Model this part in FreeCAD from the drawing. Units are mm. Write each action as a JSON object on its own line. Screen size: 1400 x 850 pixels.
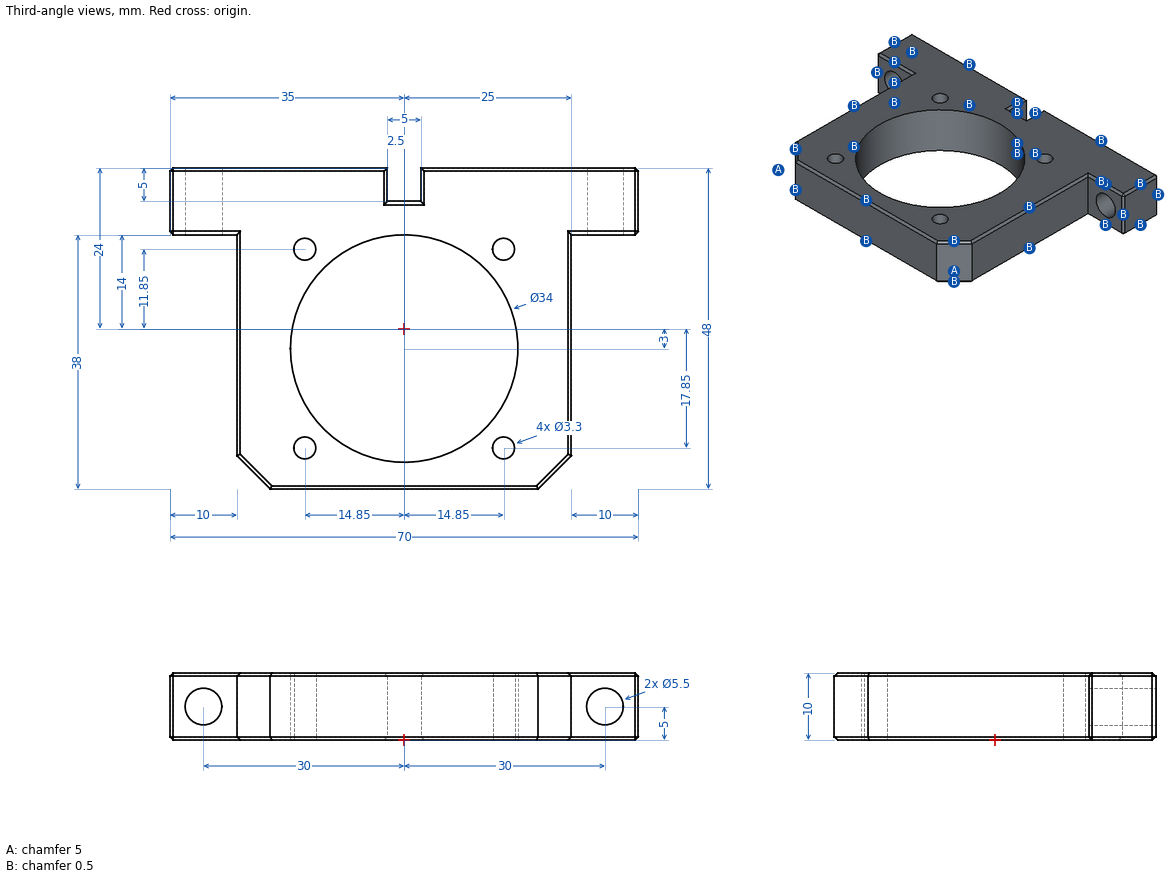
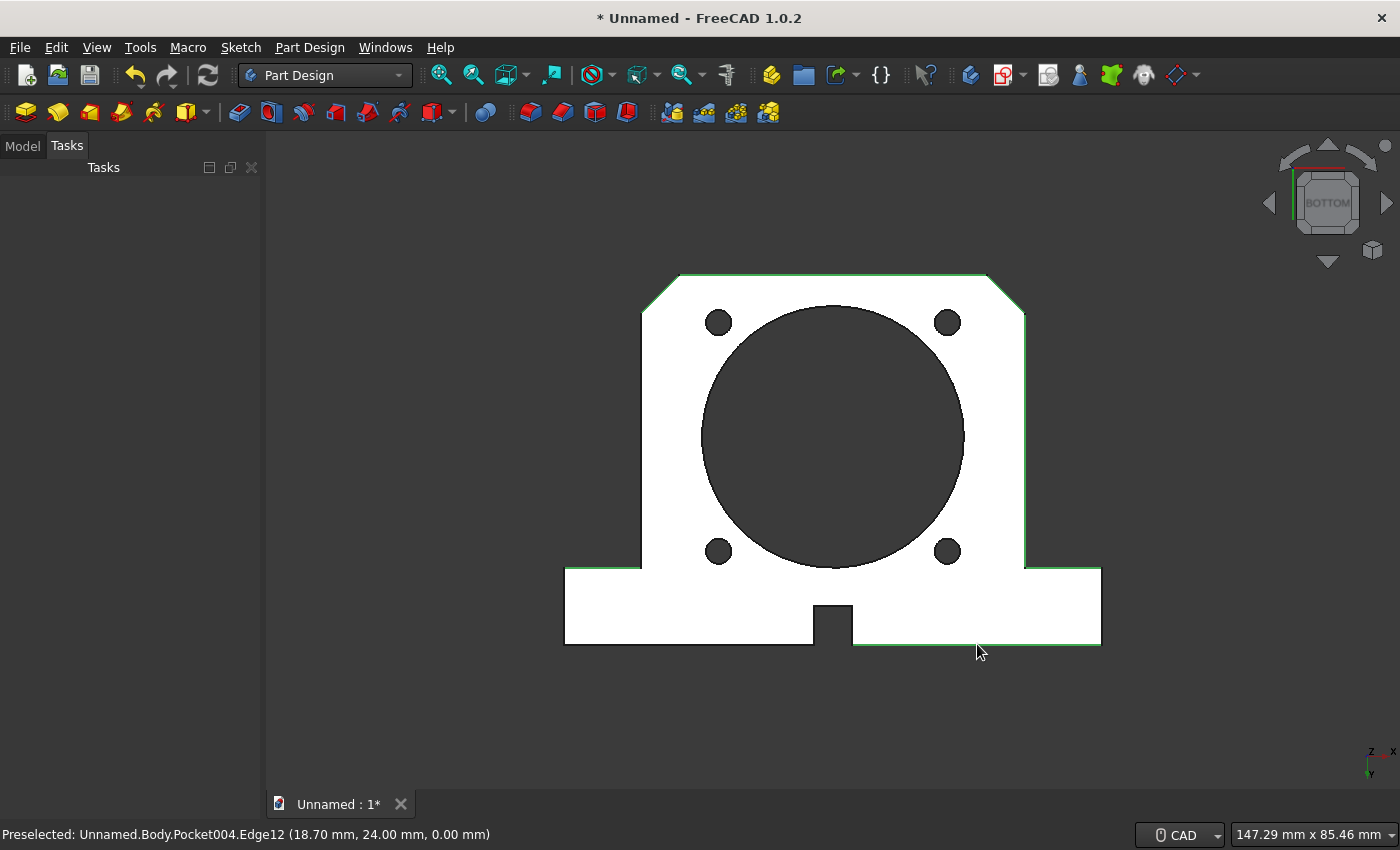
{"action": "left_click", "coordinate": [641, 440], "text": "ctrl"}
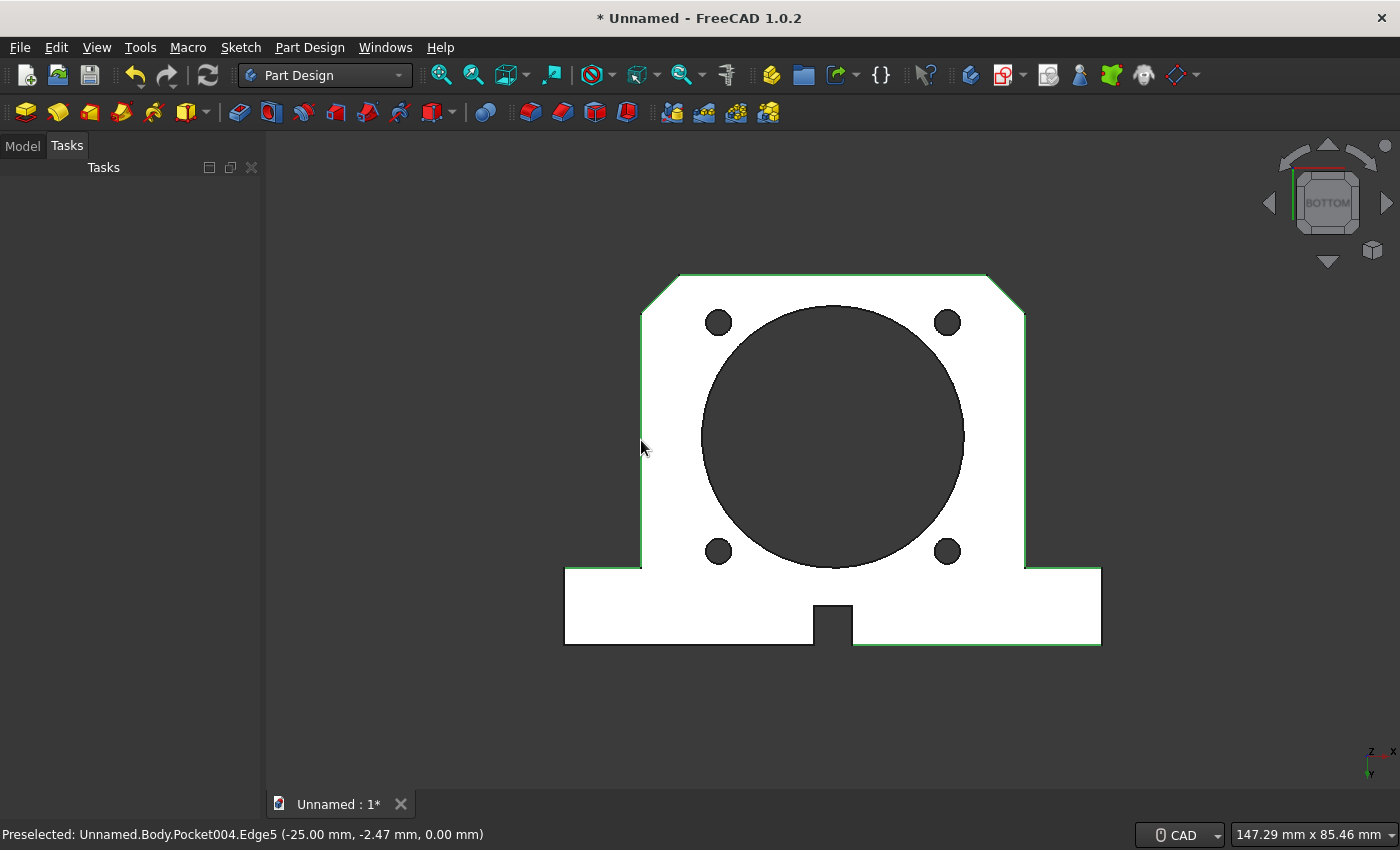
{"action": "left_click", "coordinate": [689, 644], "text": "ctrl"}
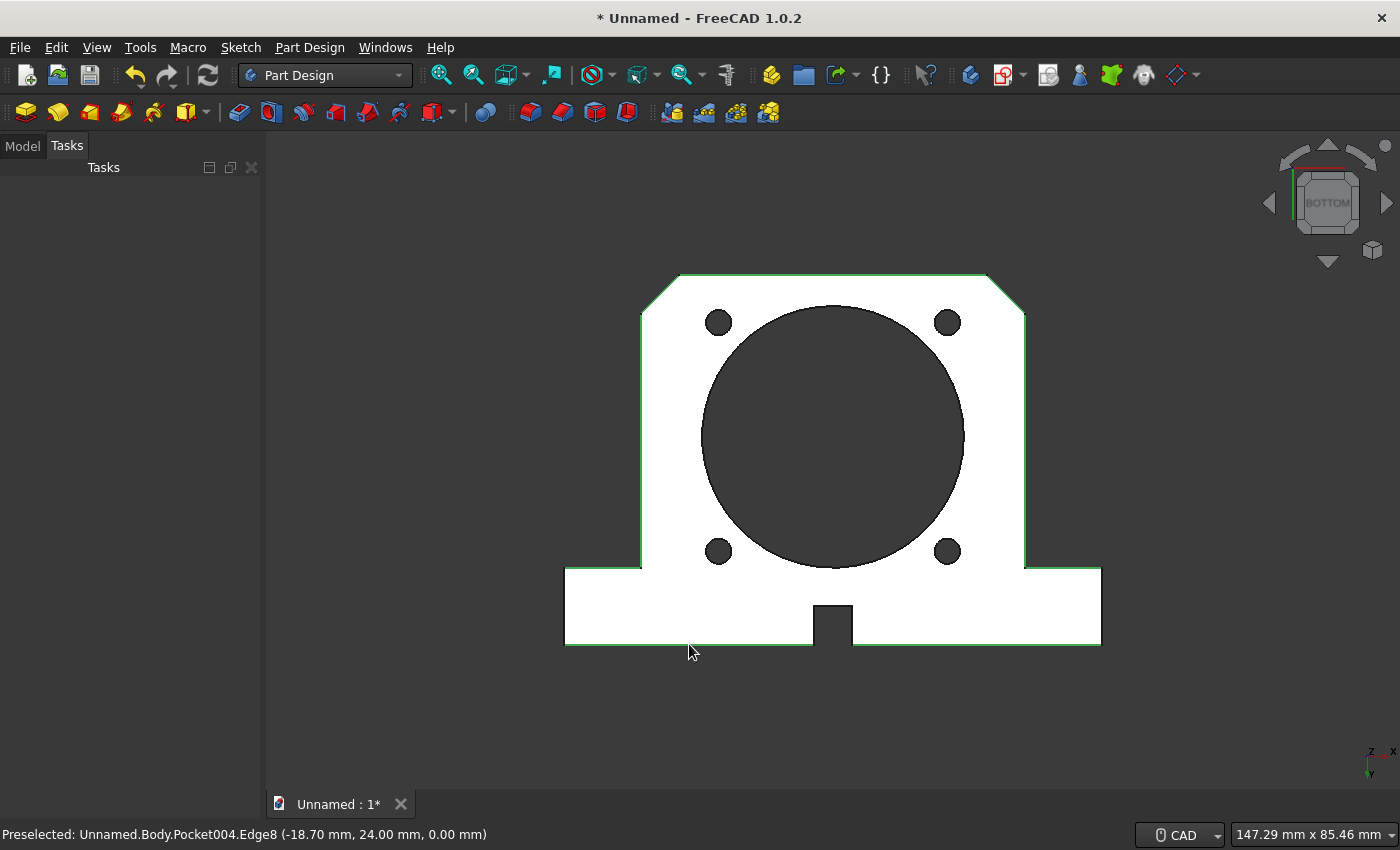
{"action": "left_click", "coordinate": [814, 625], "text": "ctrl"}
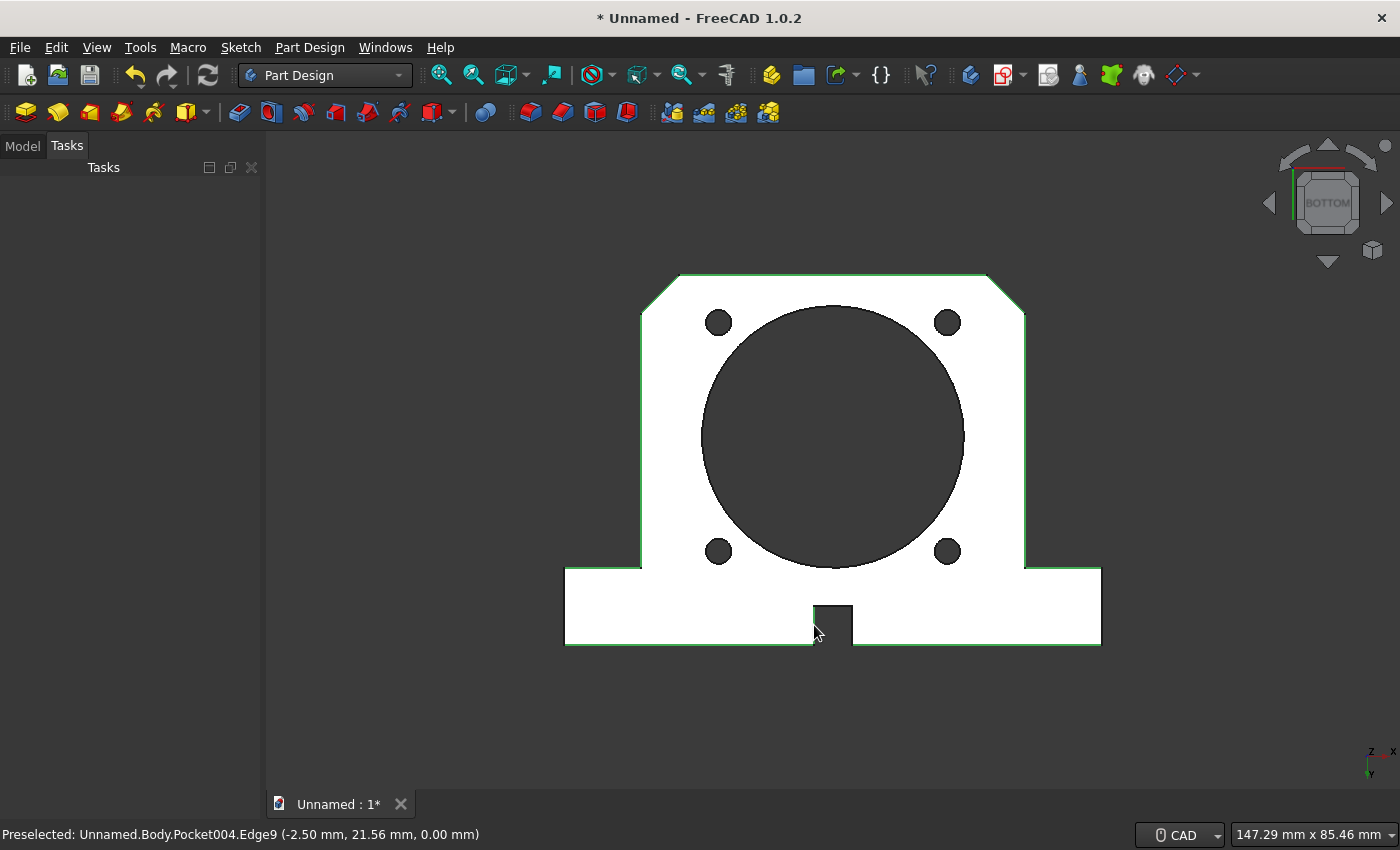
{"action": "left_click", "coordinate": [852, 625], "text": "ctrl"}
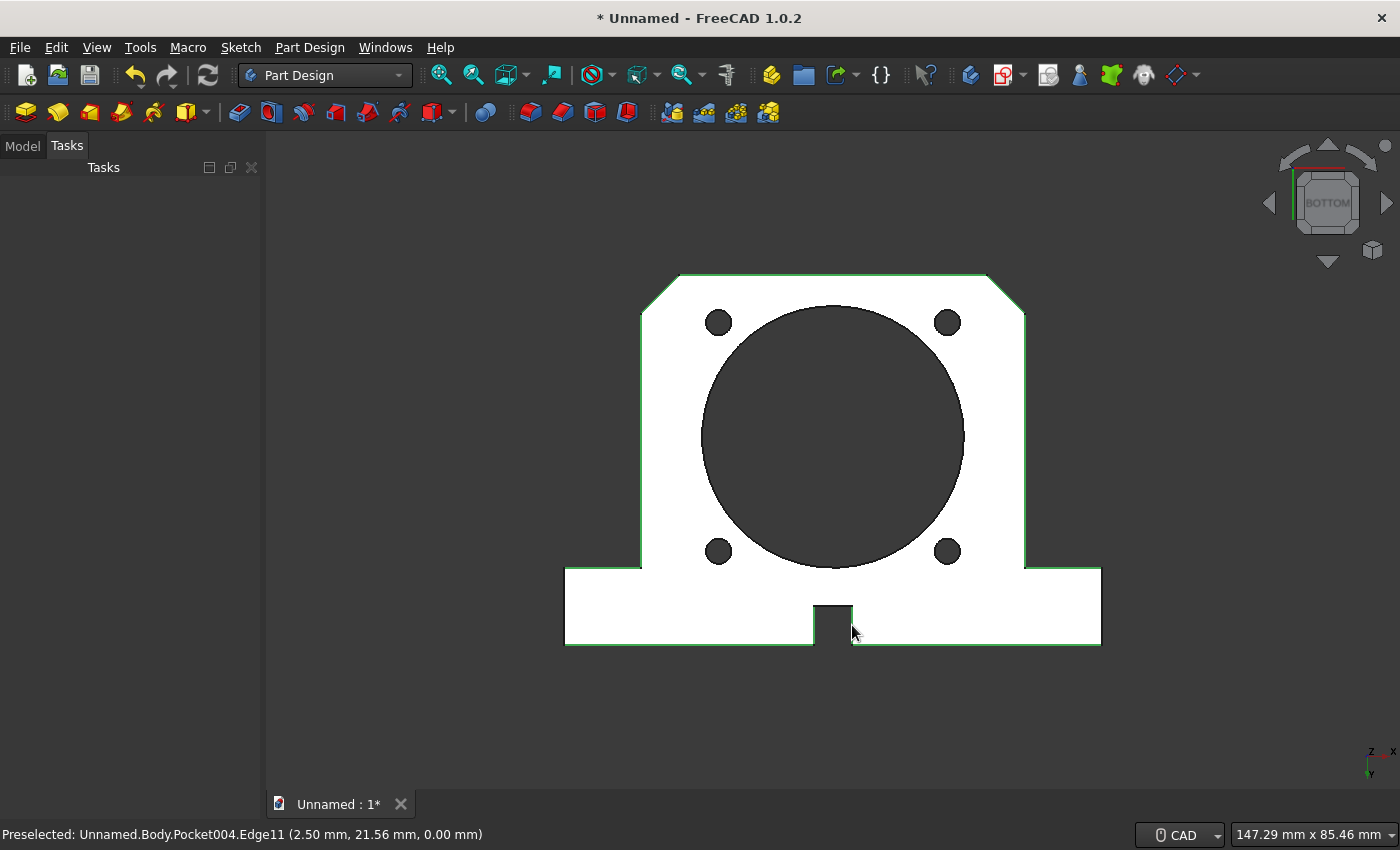
{"action": "left_click", "coordinate": [833, 605], "text": "ctrl"}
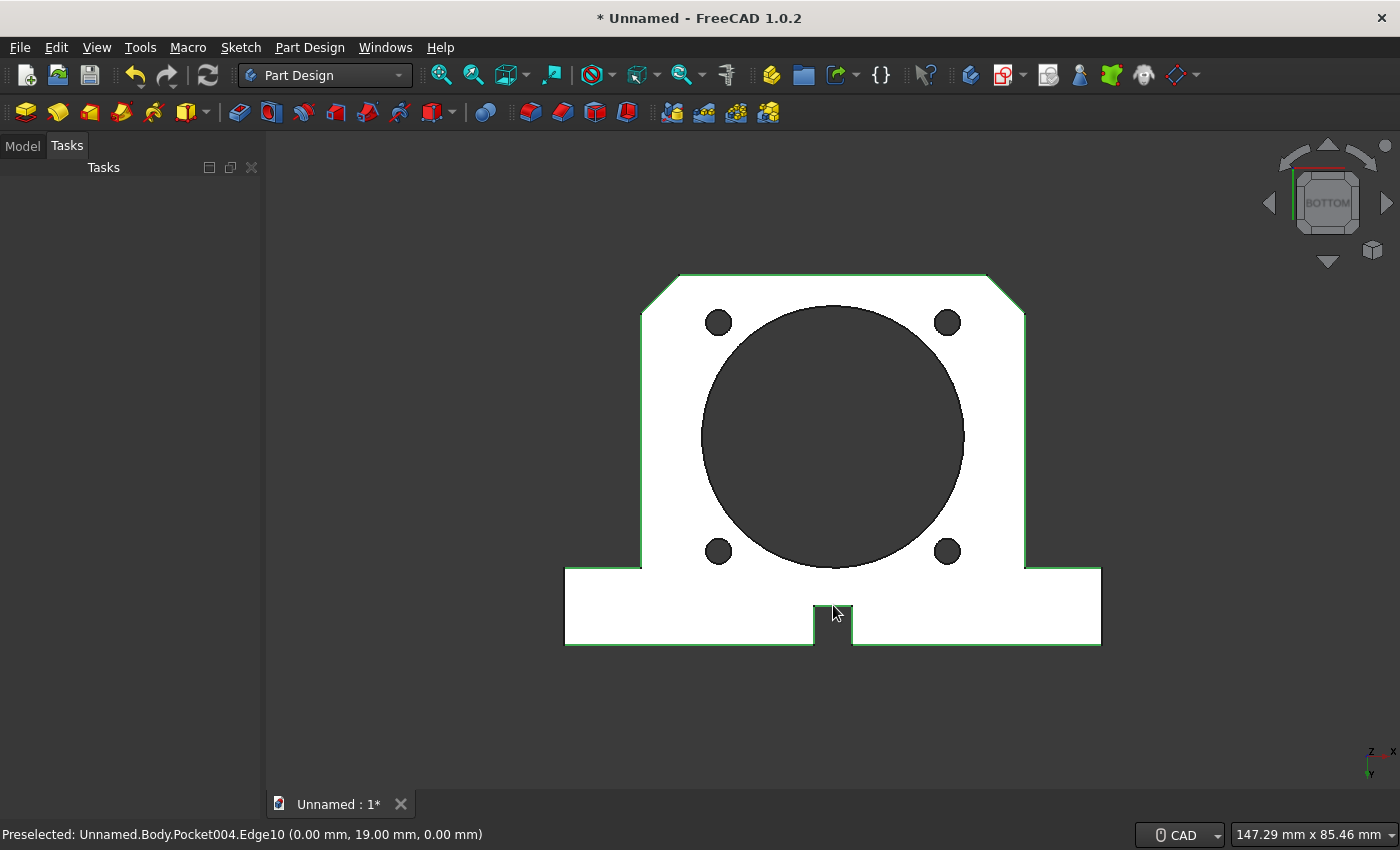
{"action": "key", "text": "4"}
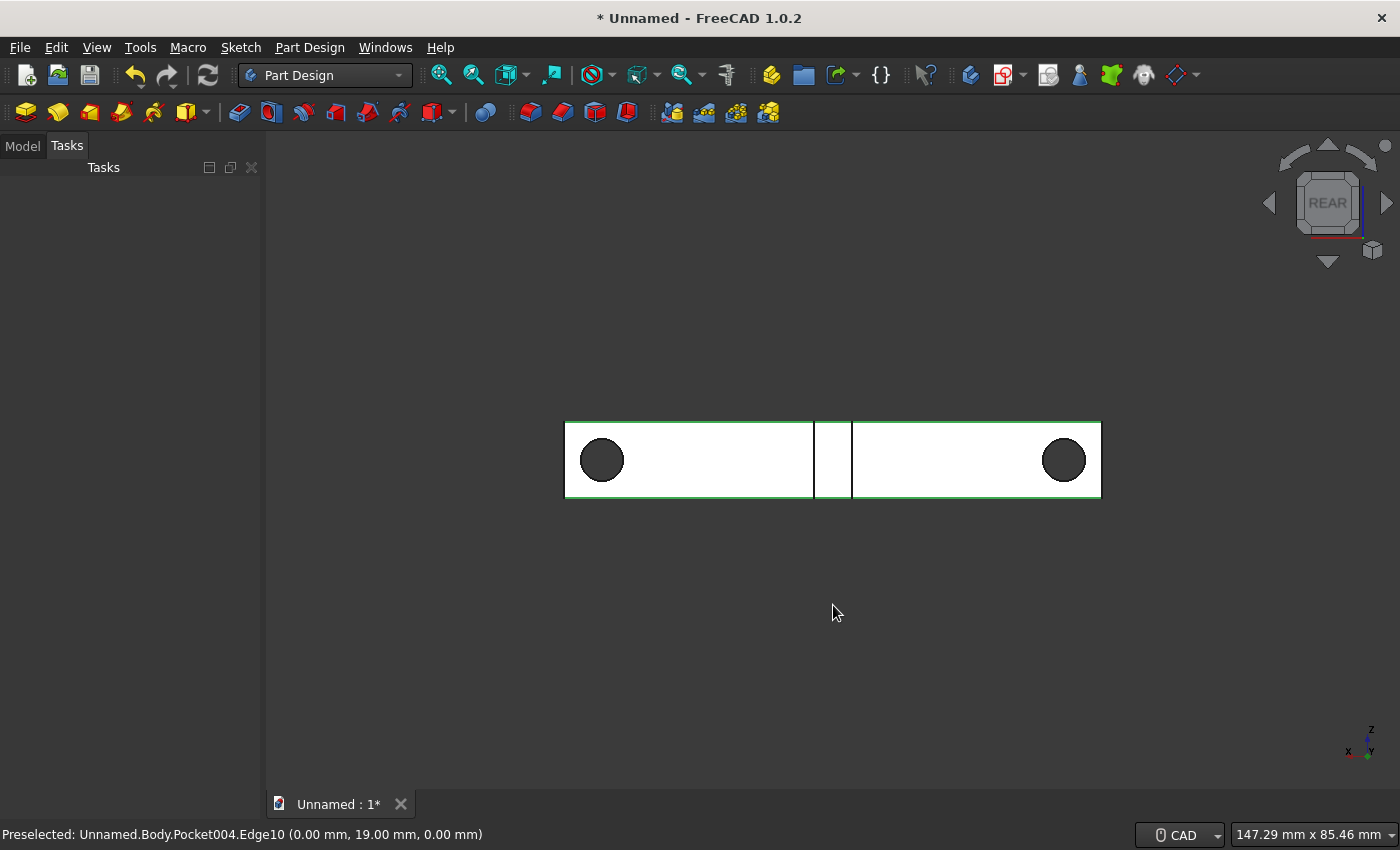
{"action": "key", "text": "6"}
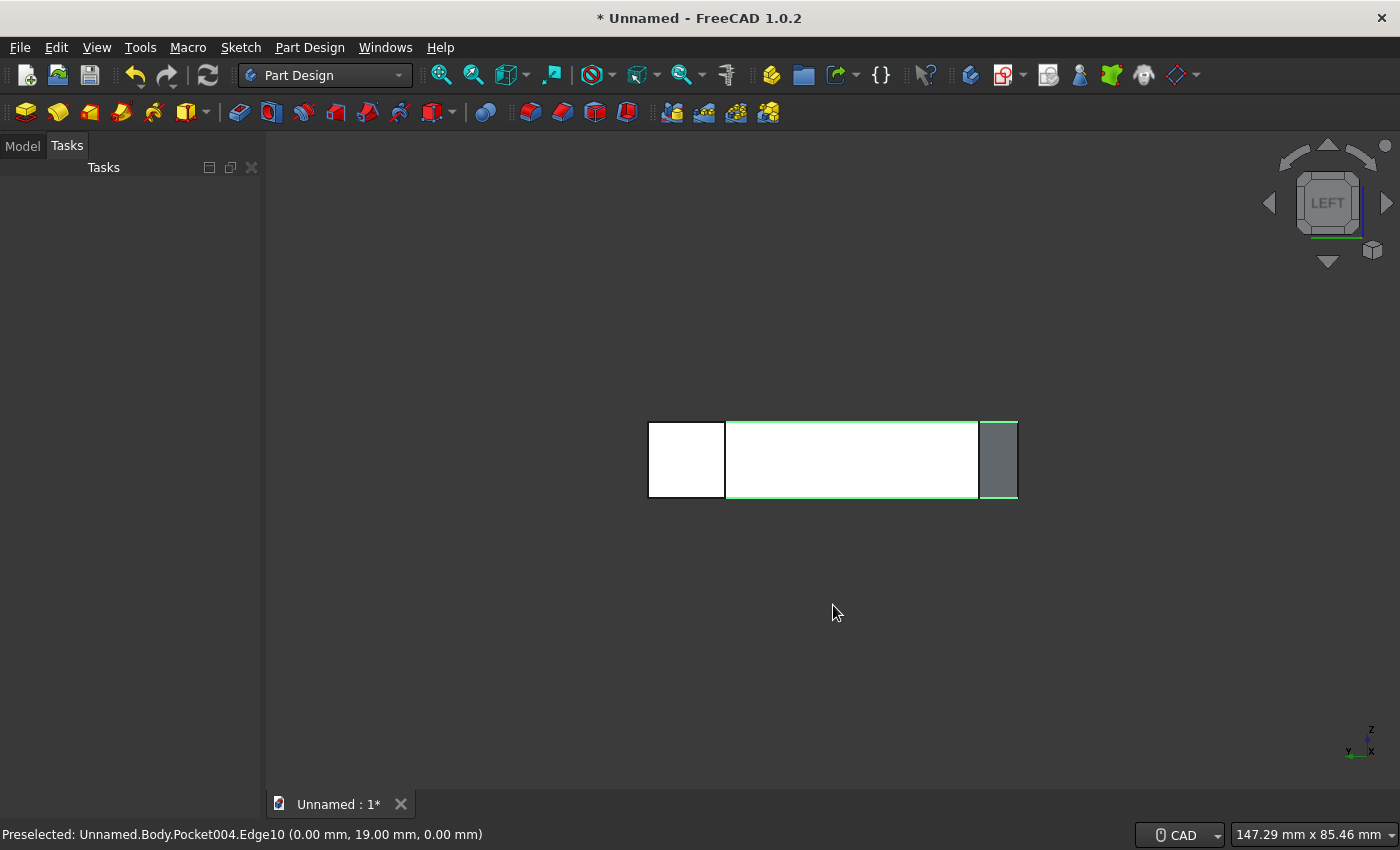
{"action": "left_click", "coordinate": [442, 76]}